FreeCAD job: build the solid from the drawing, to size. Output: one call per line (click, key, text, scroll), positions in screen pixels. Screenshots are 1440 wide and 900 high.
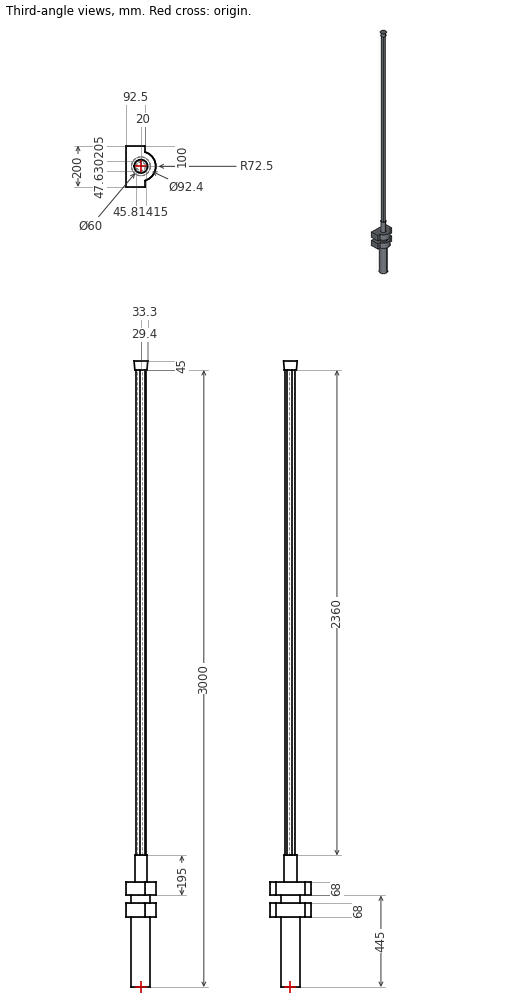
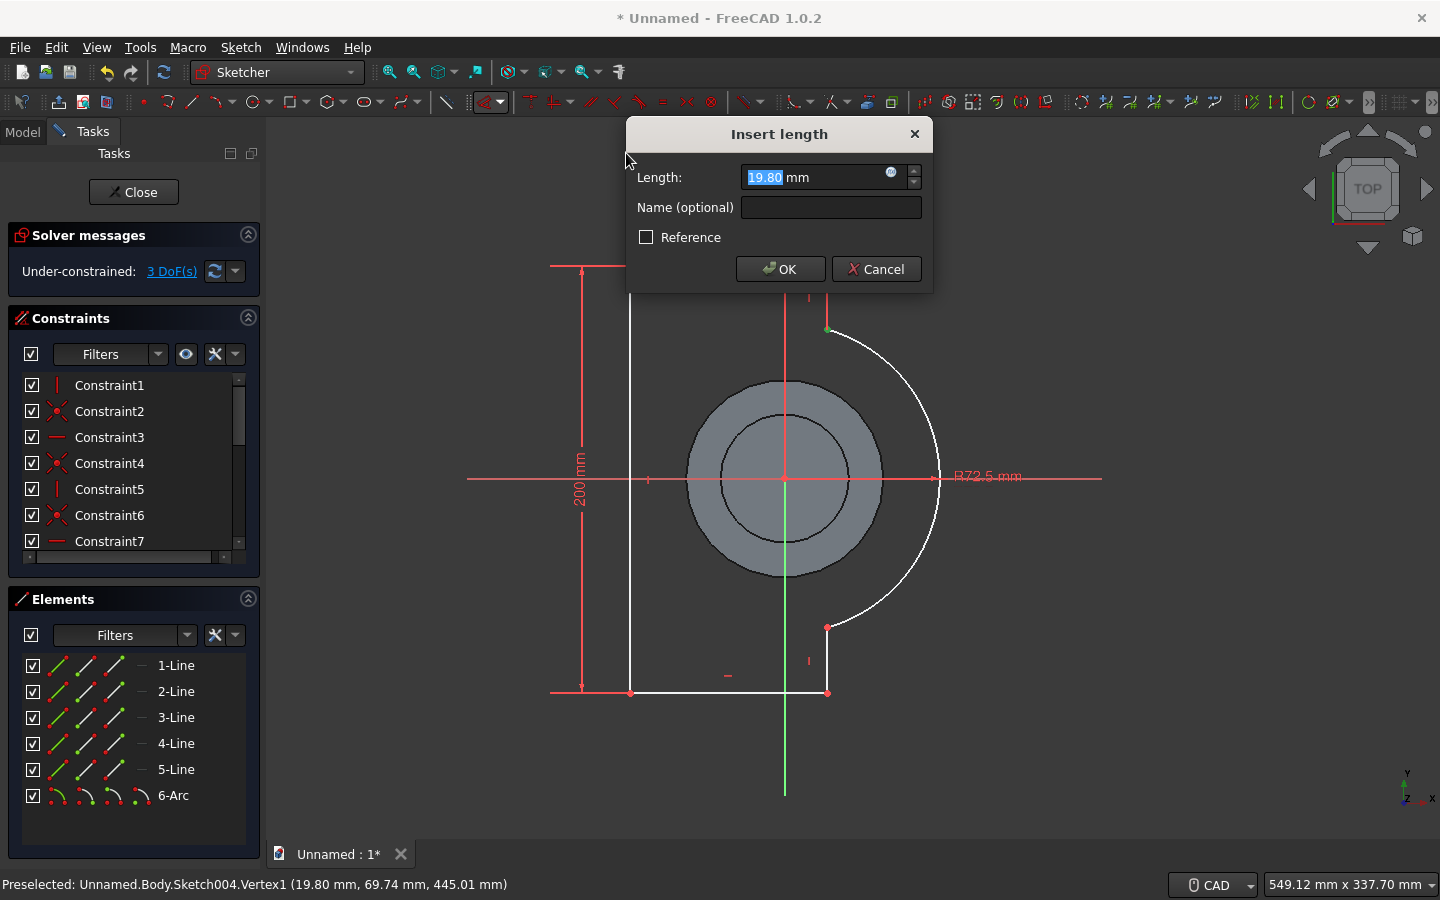
text(20)
key(Return)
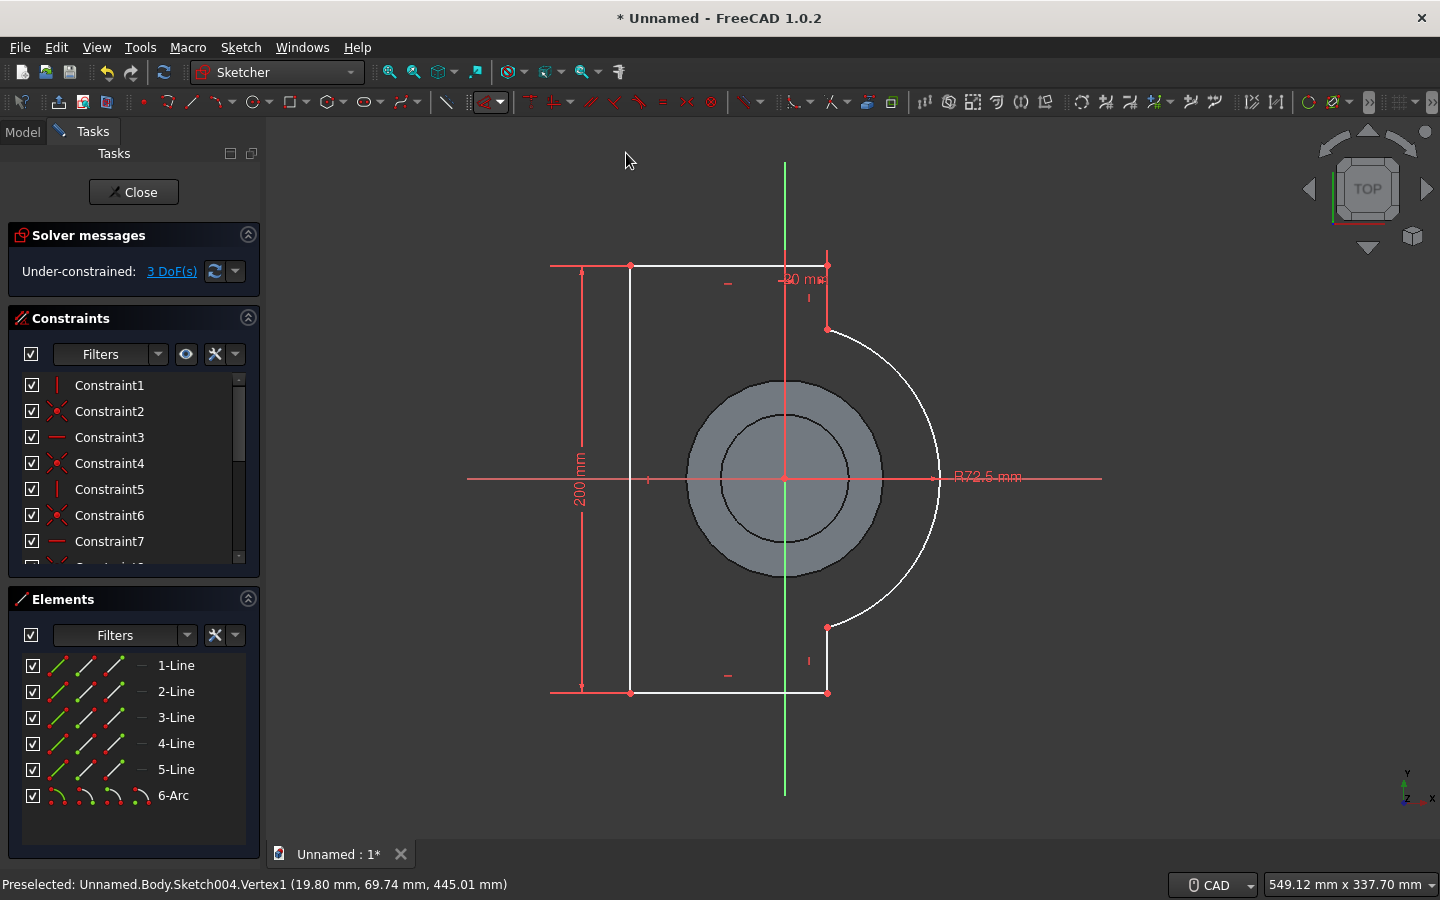
click(827, 693)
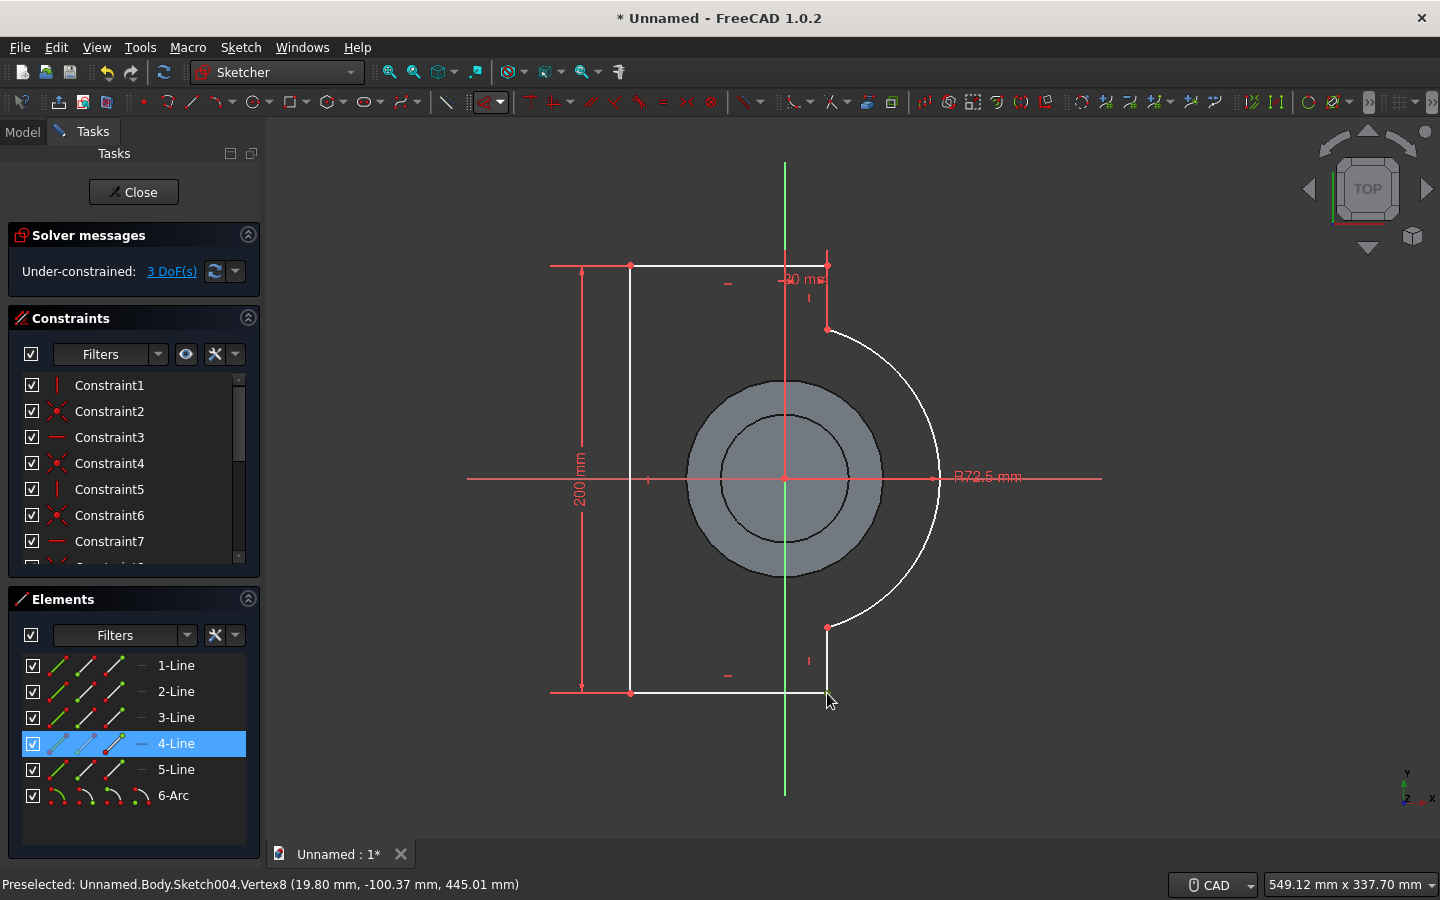
key(l)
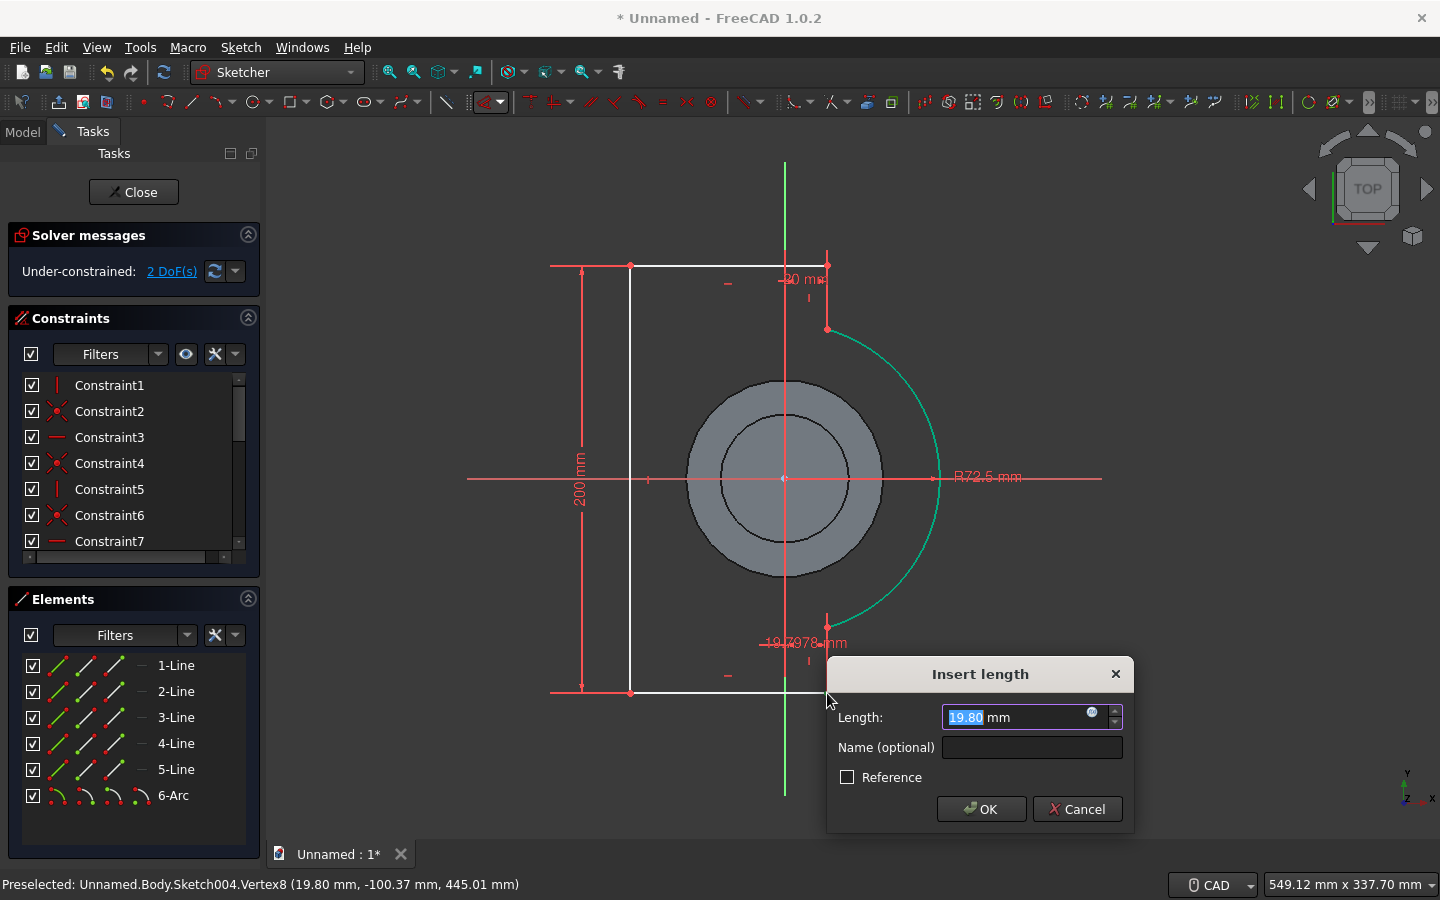
text(20)
key(Return)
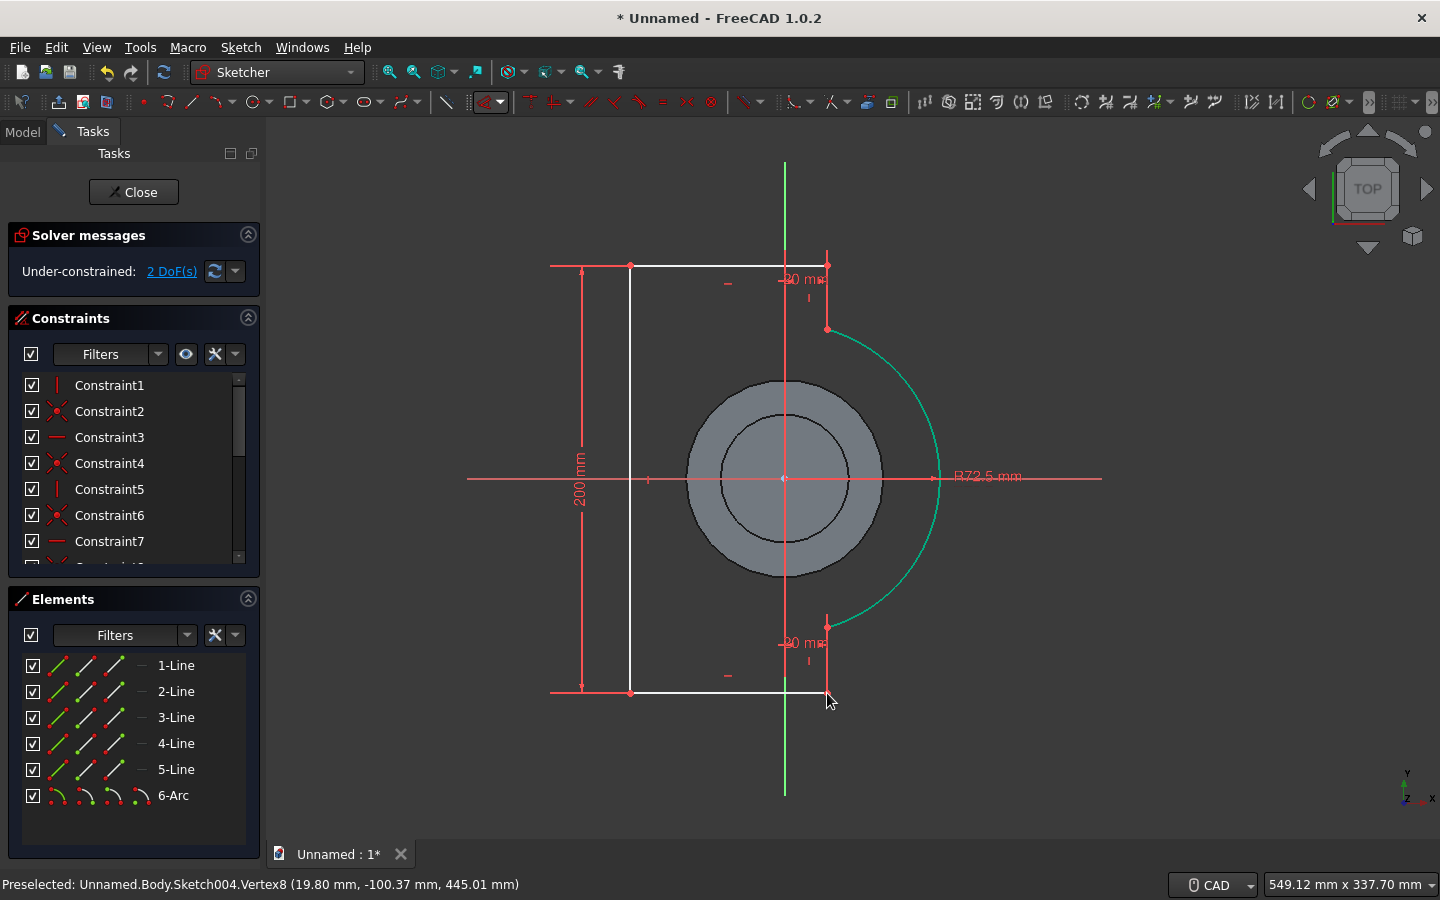
click(768, 266)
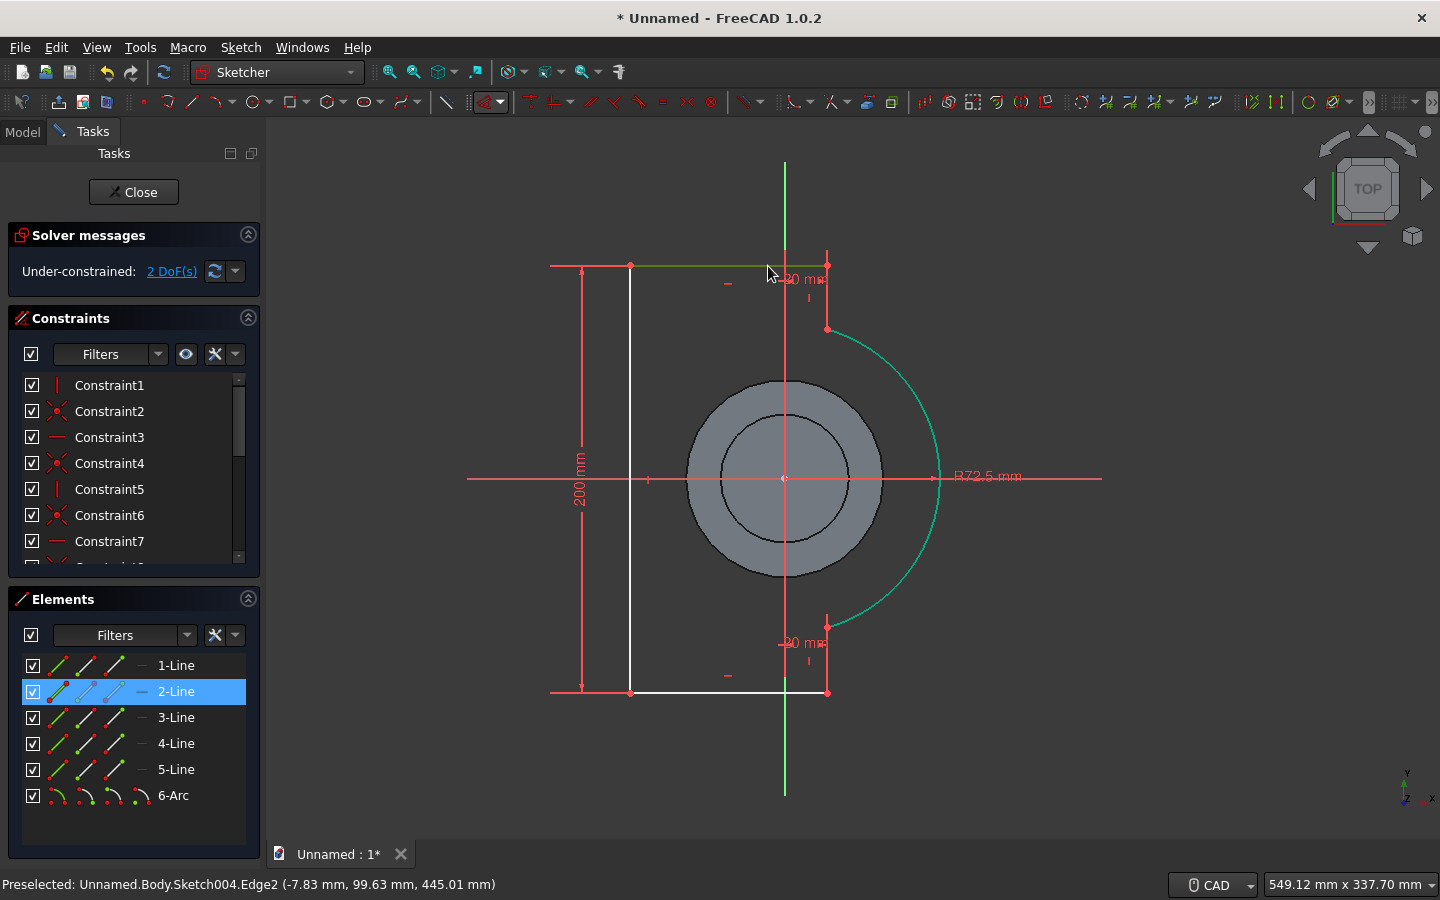
key(l)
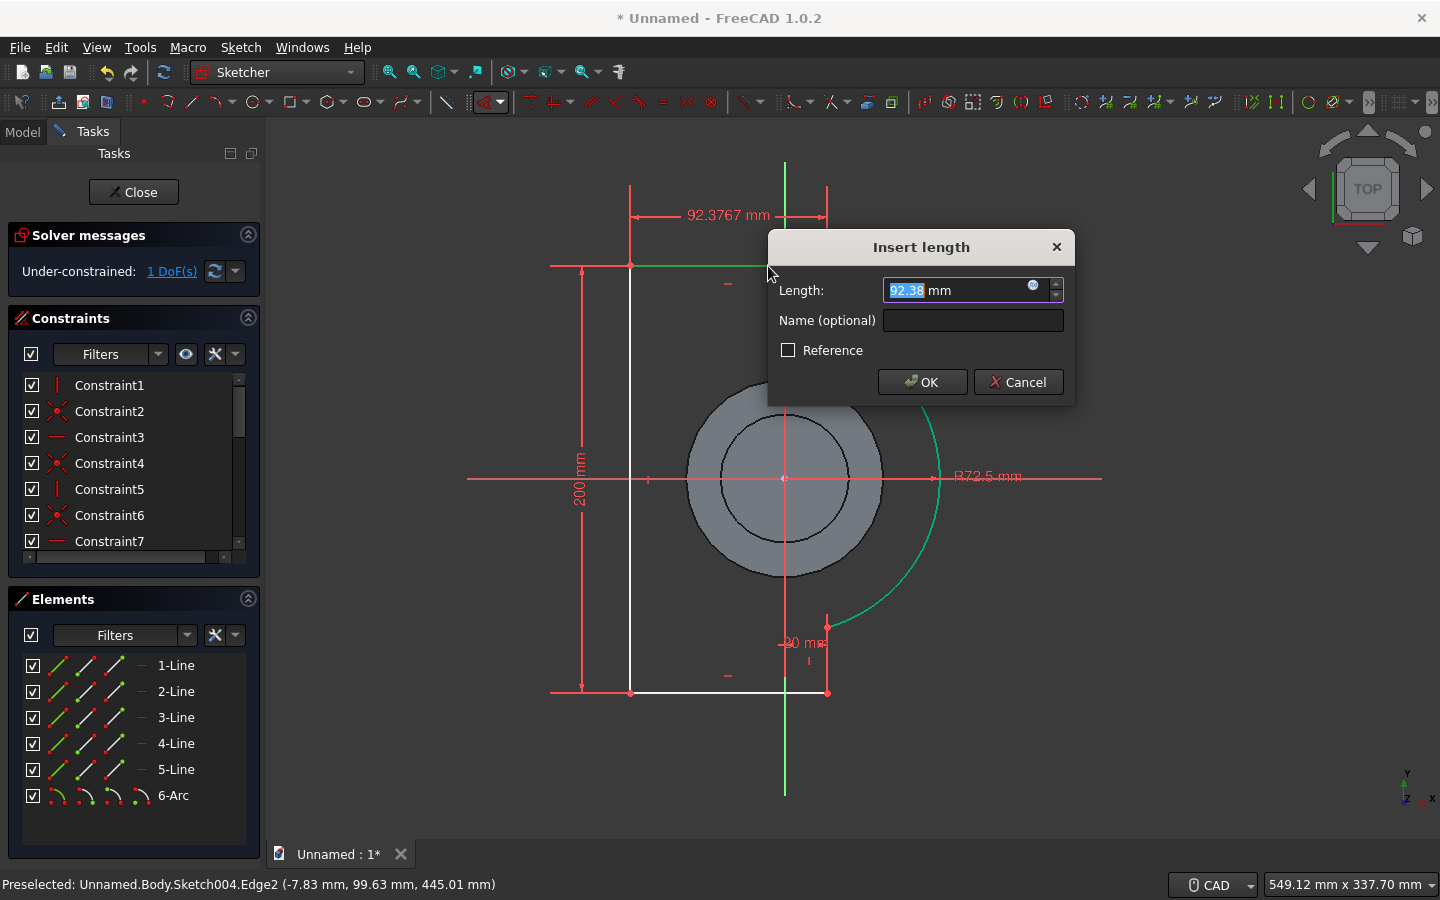
text(92.5)
key(Return)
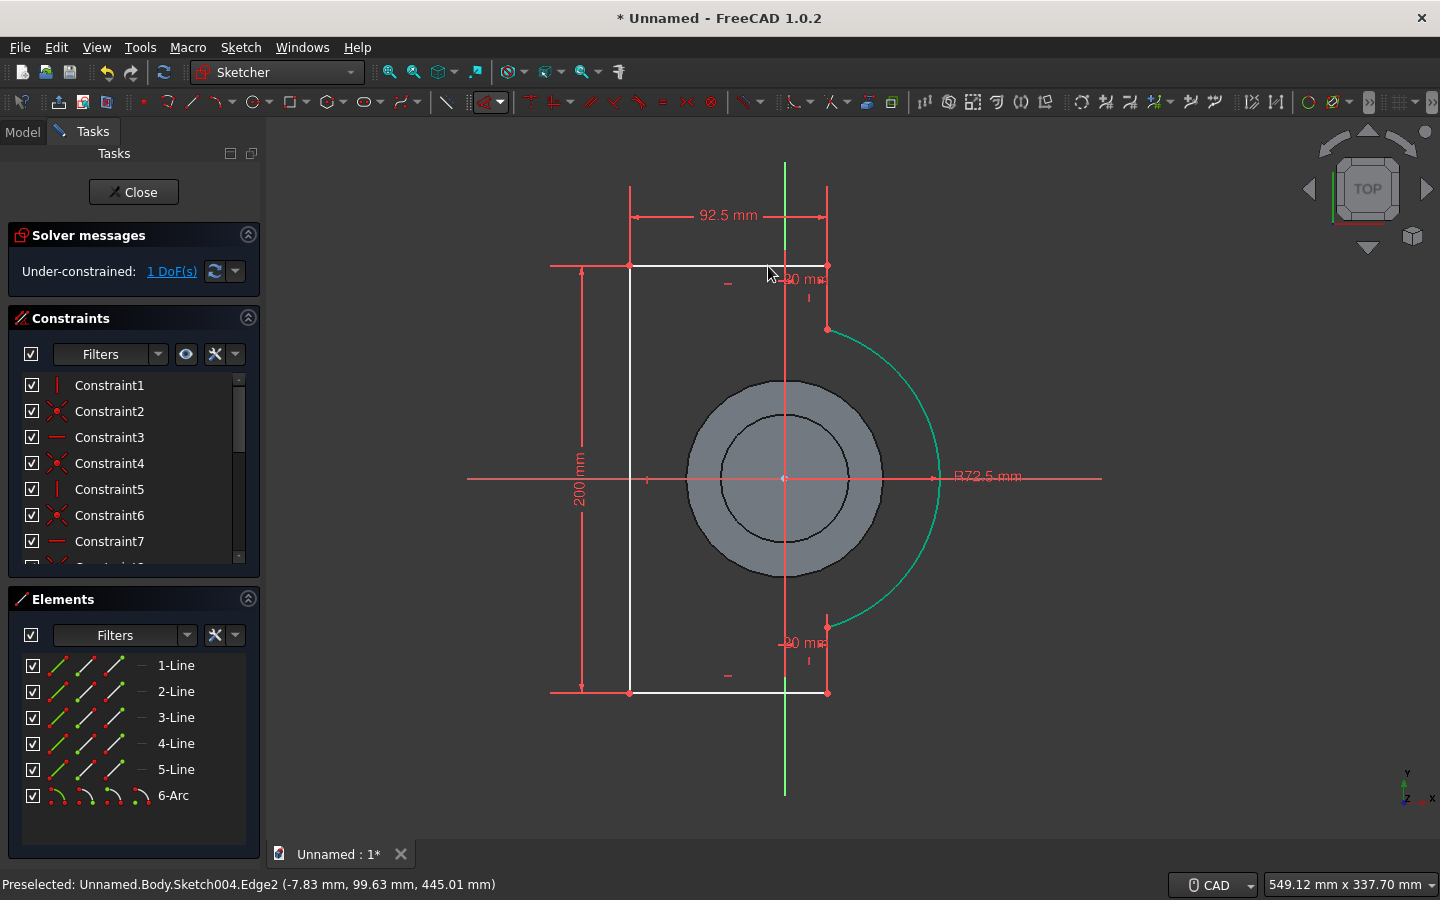
click(827, 266)